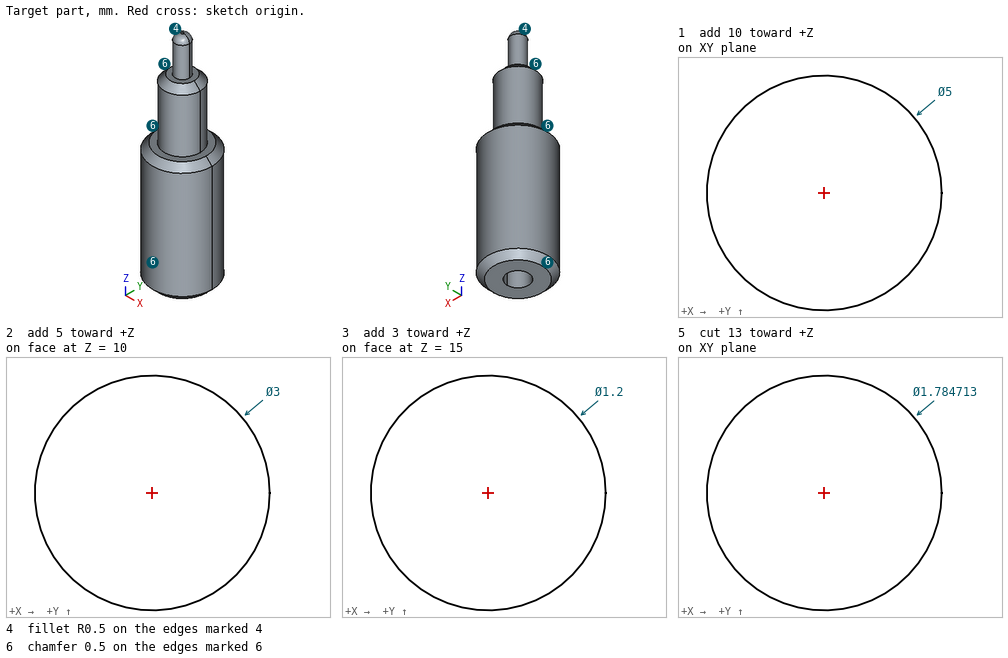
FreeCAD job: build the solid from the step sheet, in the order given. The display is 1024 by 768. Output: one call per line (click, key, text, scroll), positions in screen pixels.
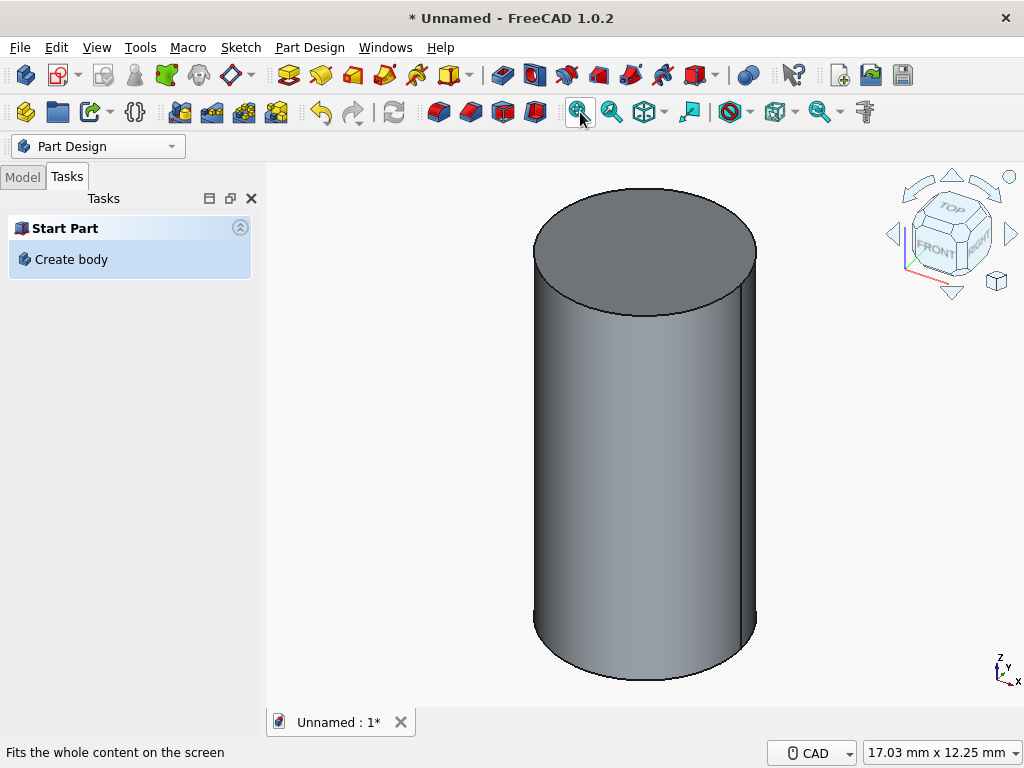
click(645, 251)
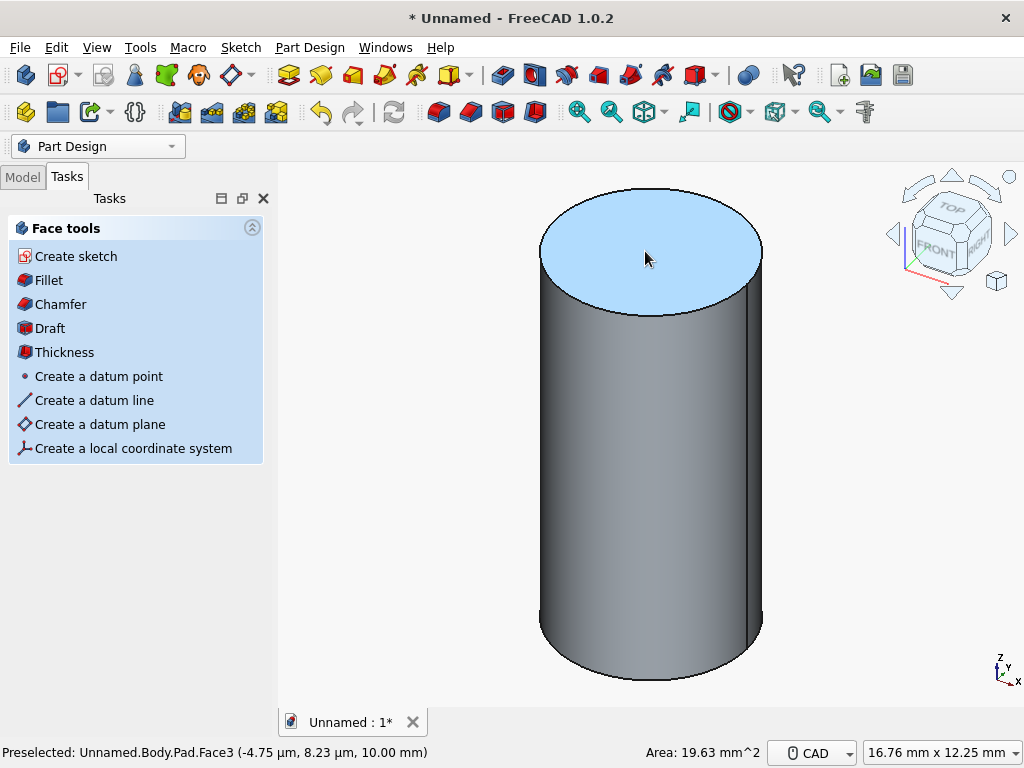
click(58, 76)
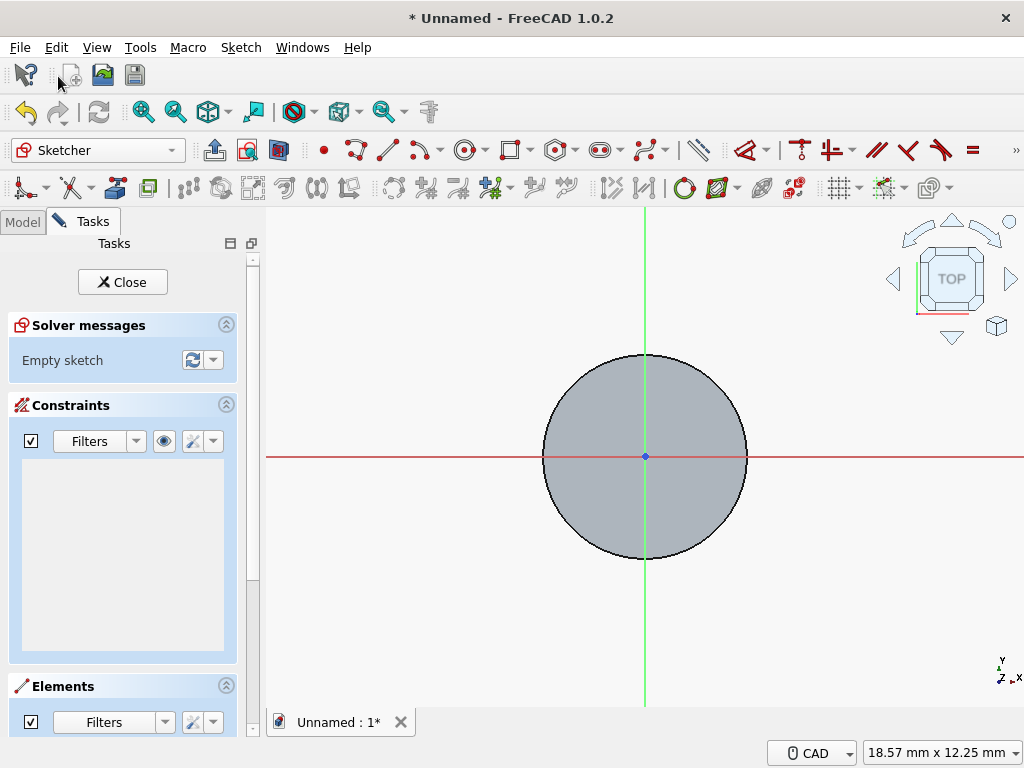
scroll(685, 457, up, 5)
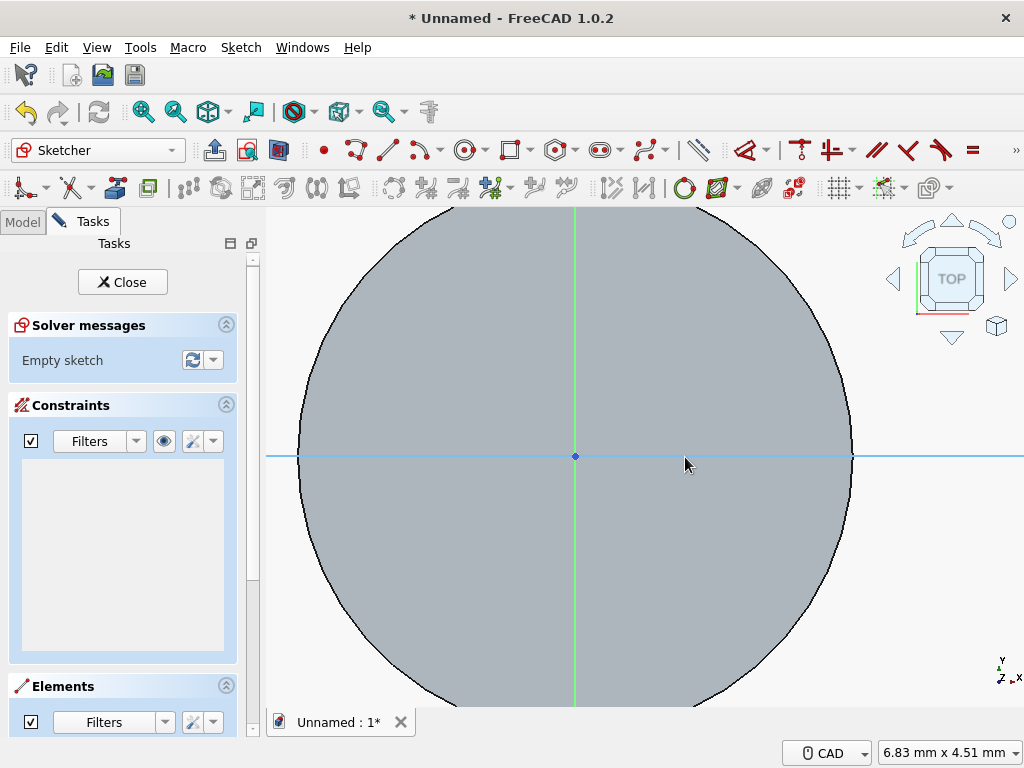
click(466, 150)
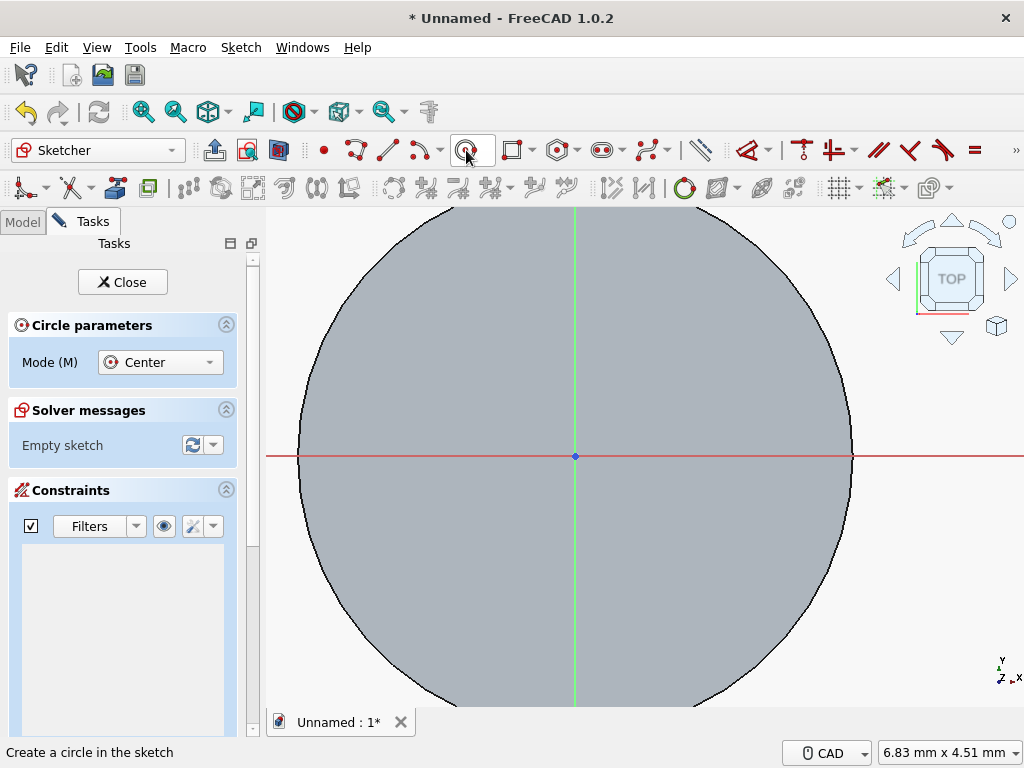
click(575, 456)
move(693, 338)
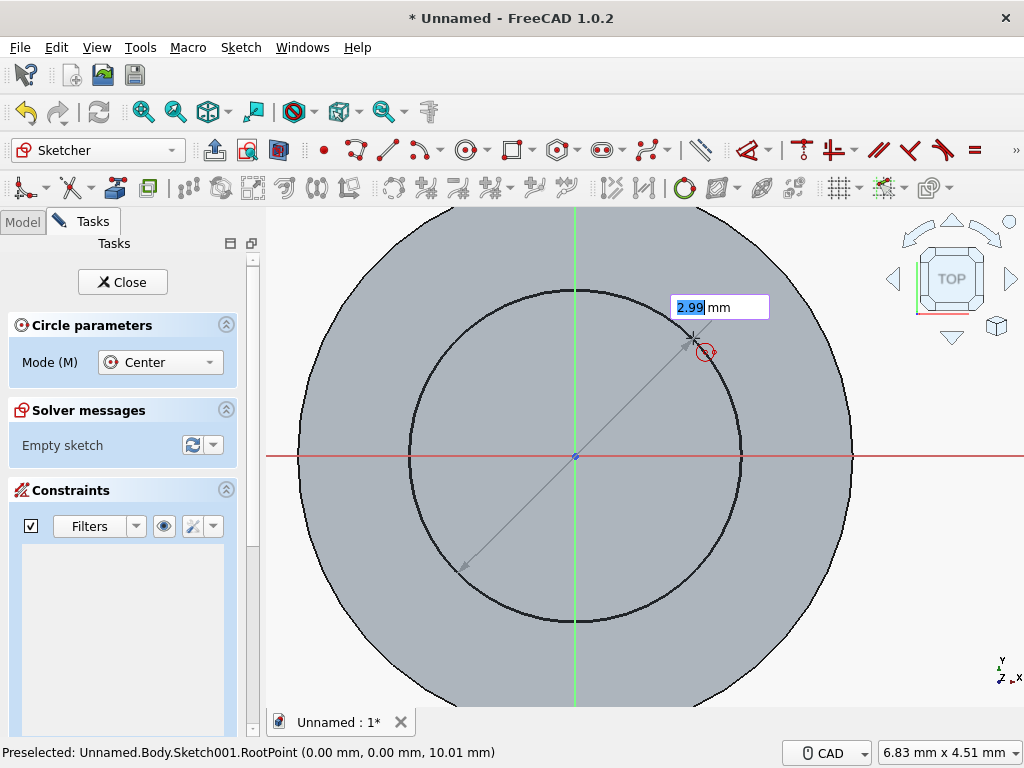
text(3)
key(Return)
key(Escape)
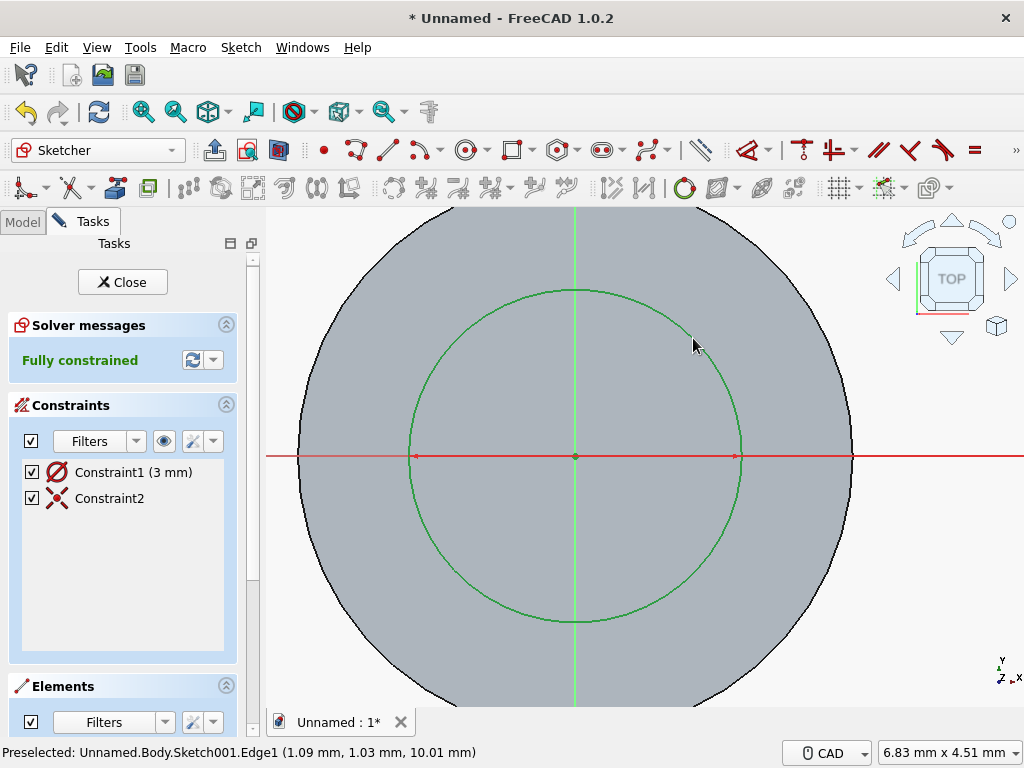
click(123, 282)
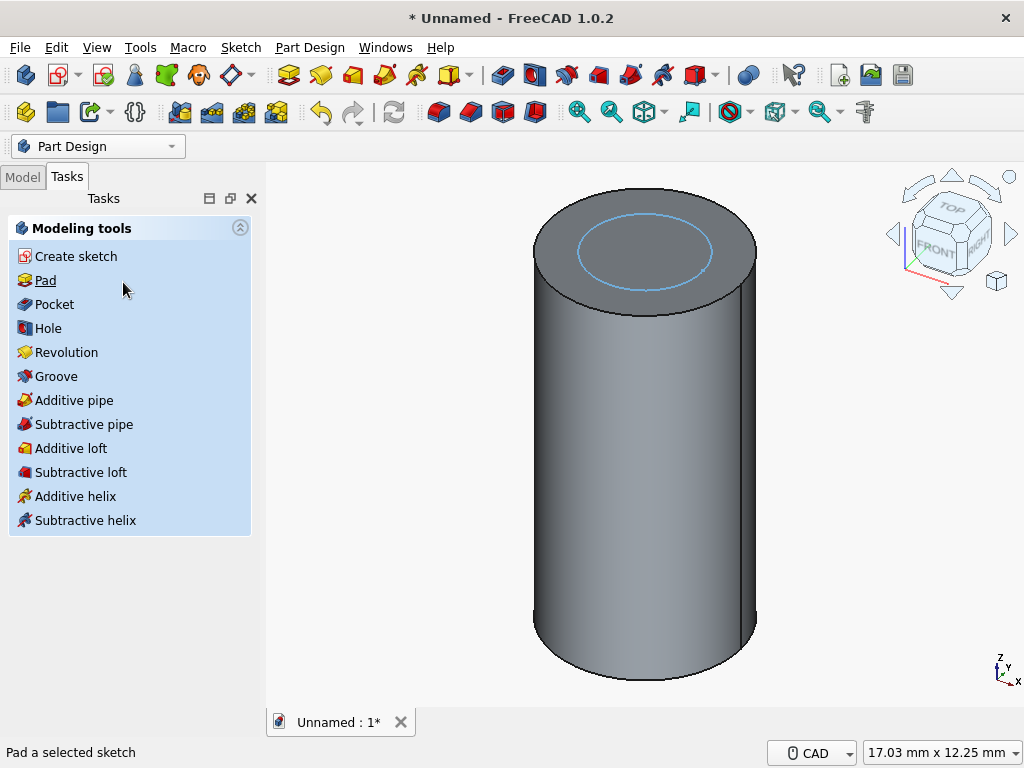
click(290, 76)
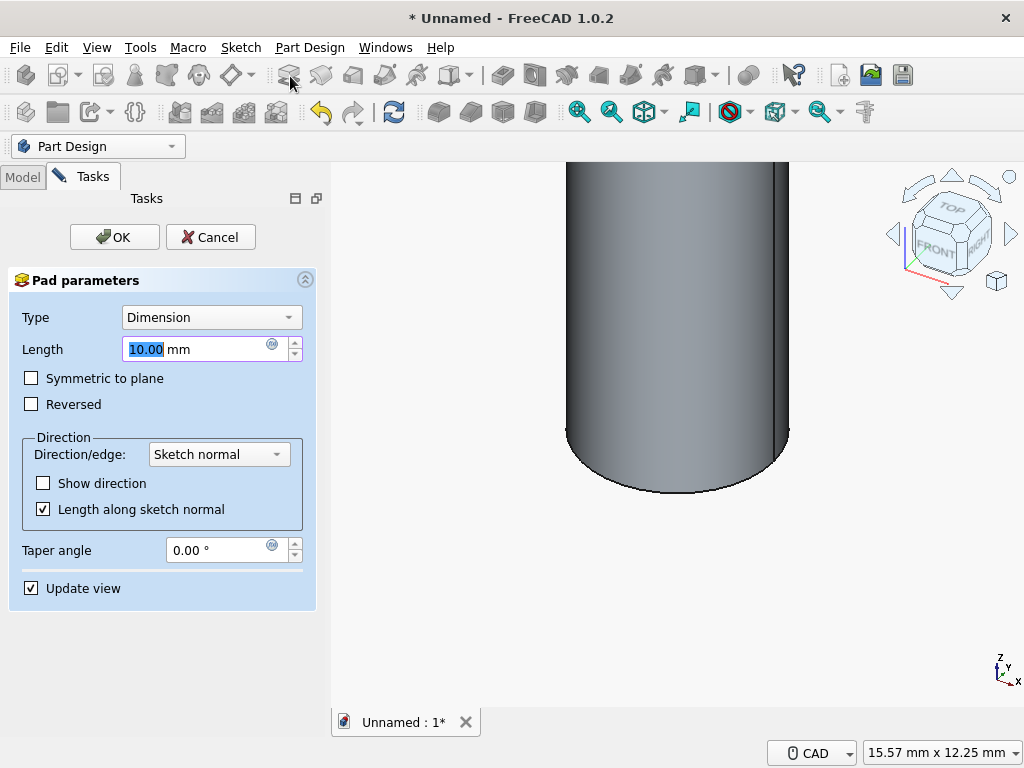
text(5)
key(Tab)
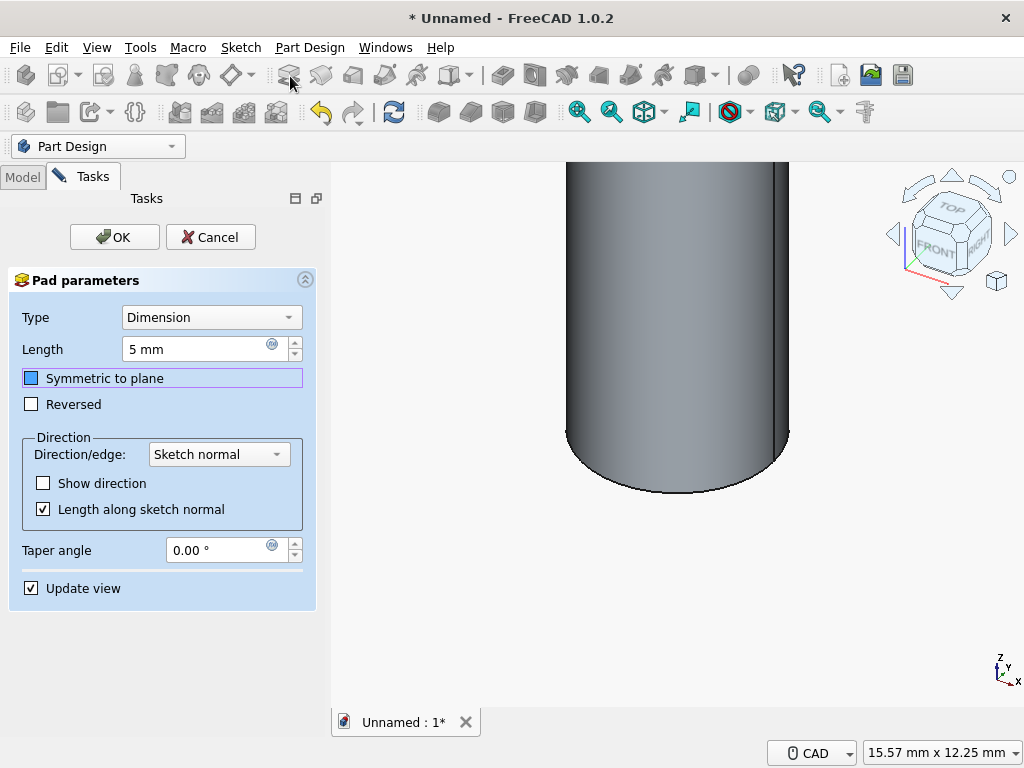
click(115, 237)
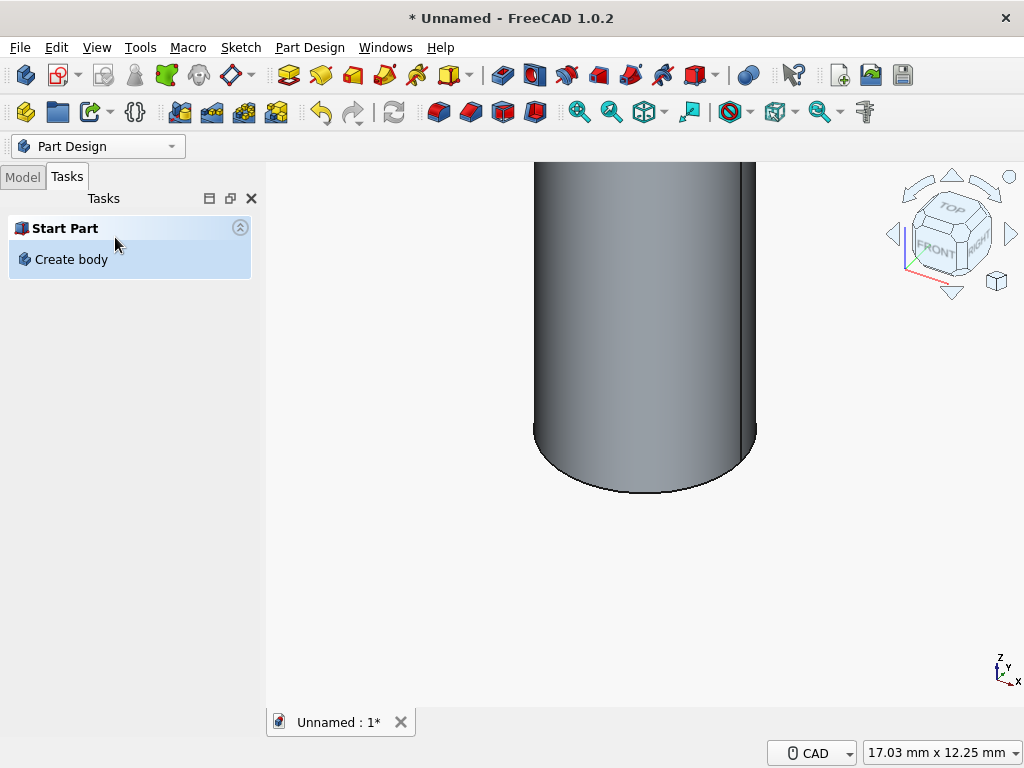
click(580, 112)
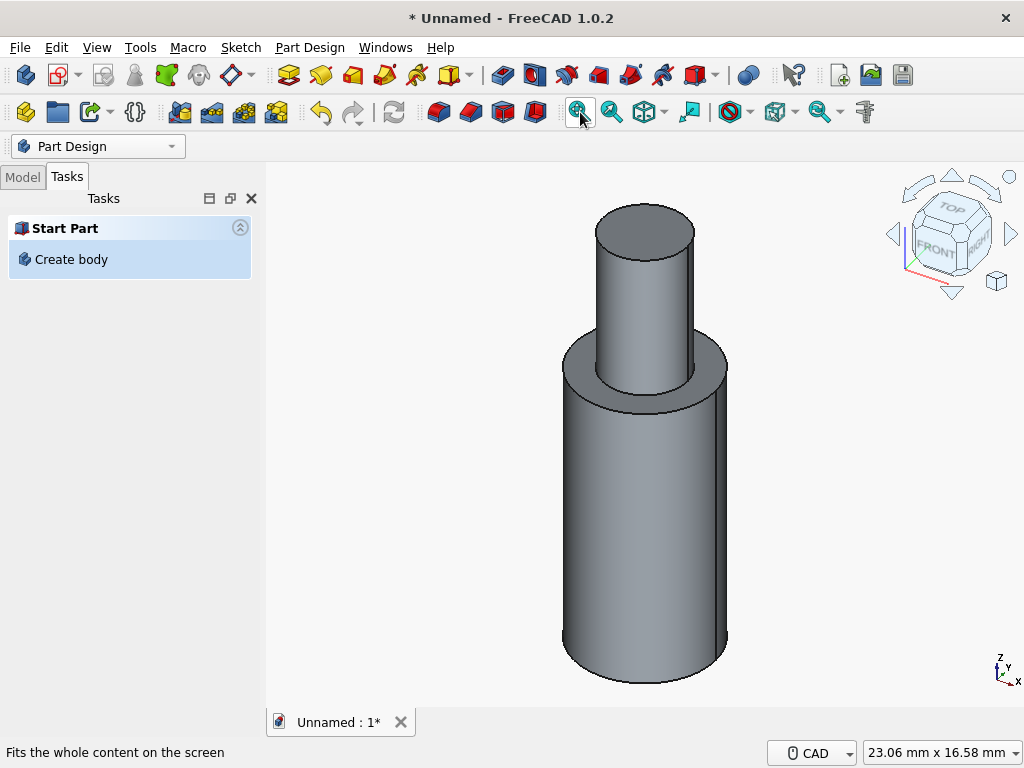
click(645, 232)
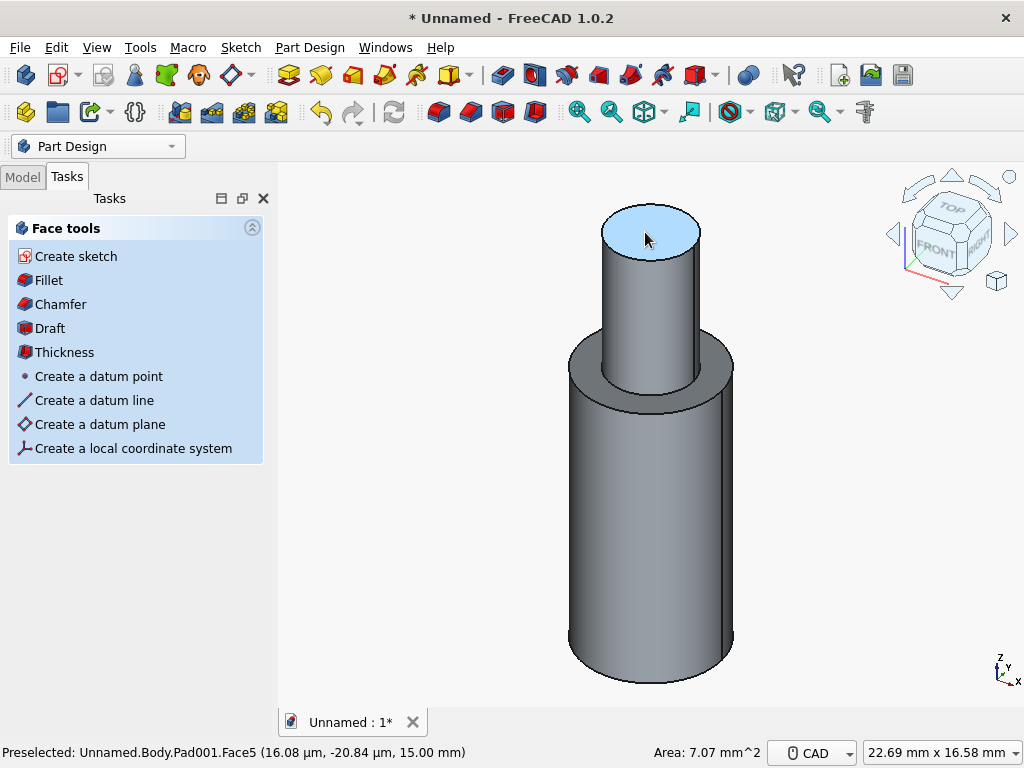
click(58, 76)